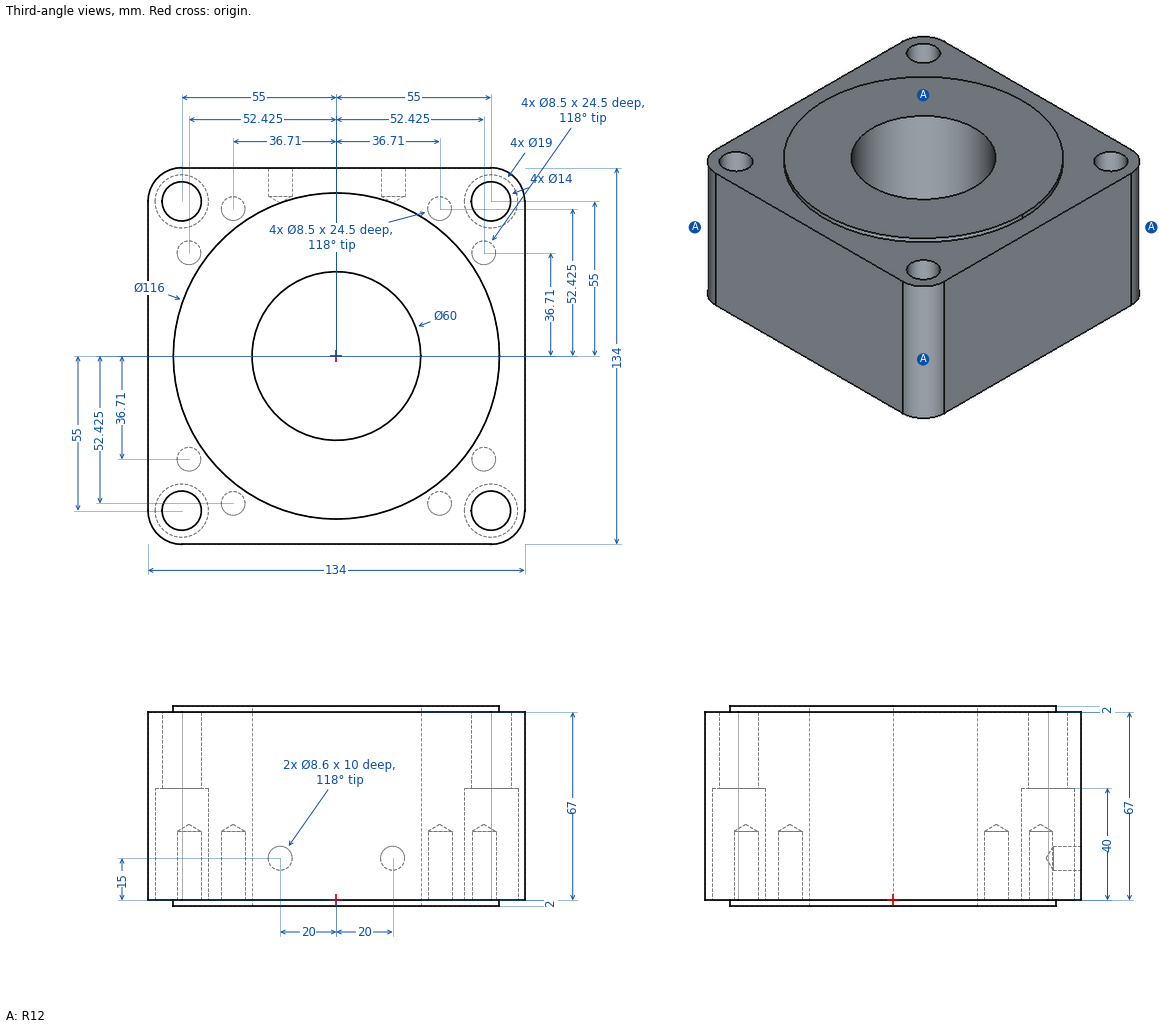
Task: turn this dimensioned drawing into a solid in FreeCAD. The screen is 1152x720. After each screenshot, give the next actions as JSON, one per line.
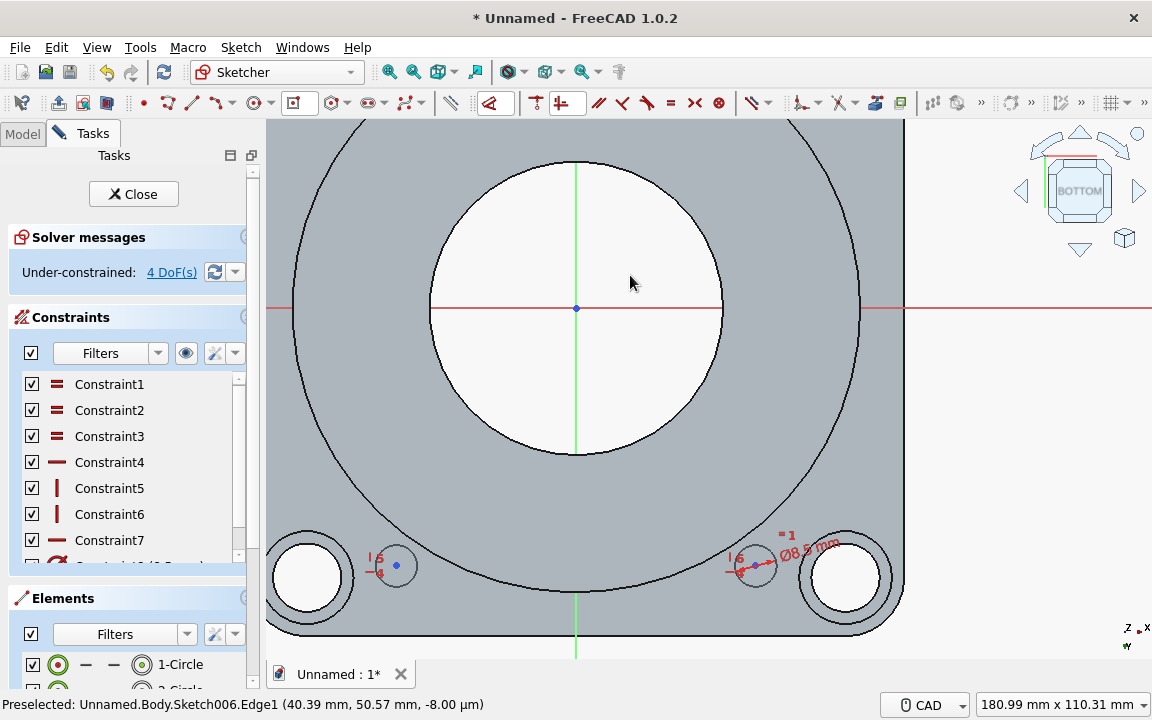
{"action": "left_click", "coordinate": [756, 566]}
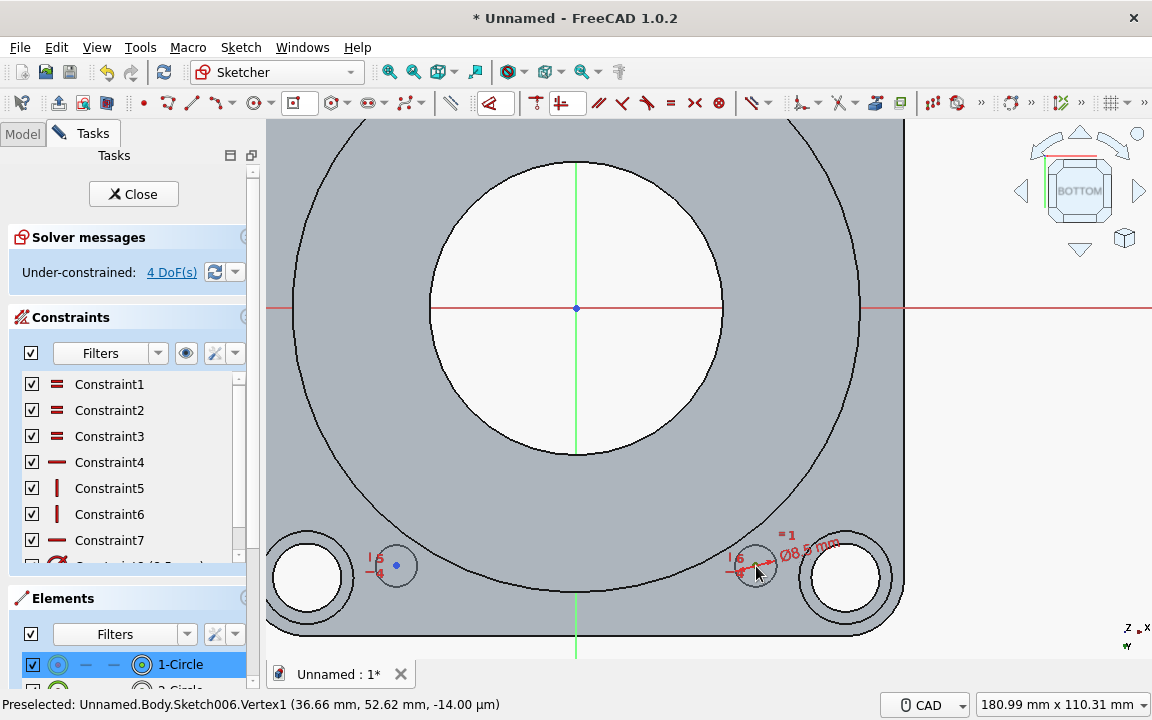
{"action": "key", "text": "l"}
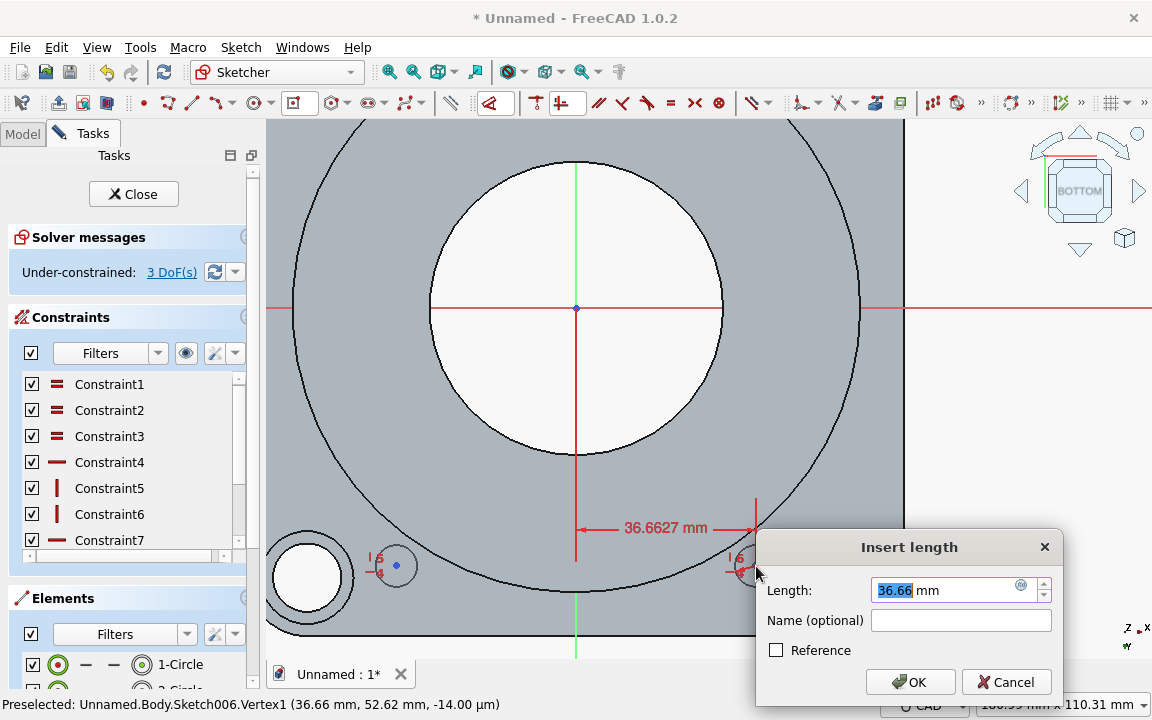
{"action": "type", "text": "36.71"}
{"action": "key", "text": "Return"}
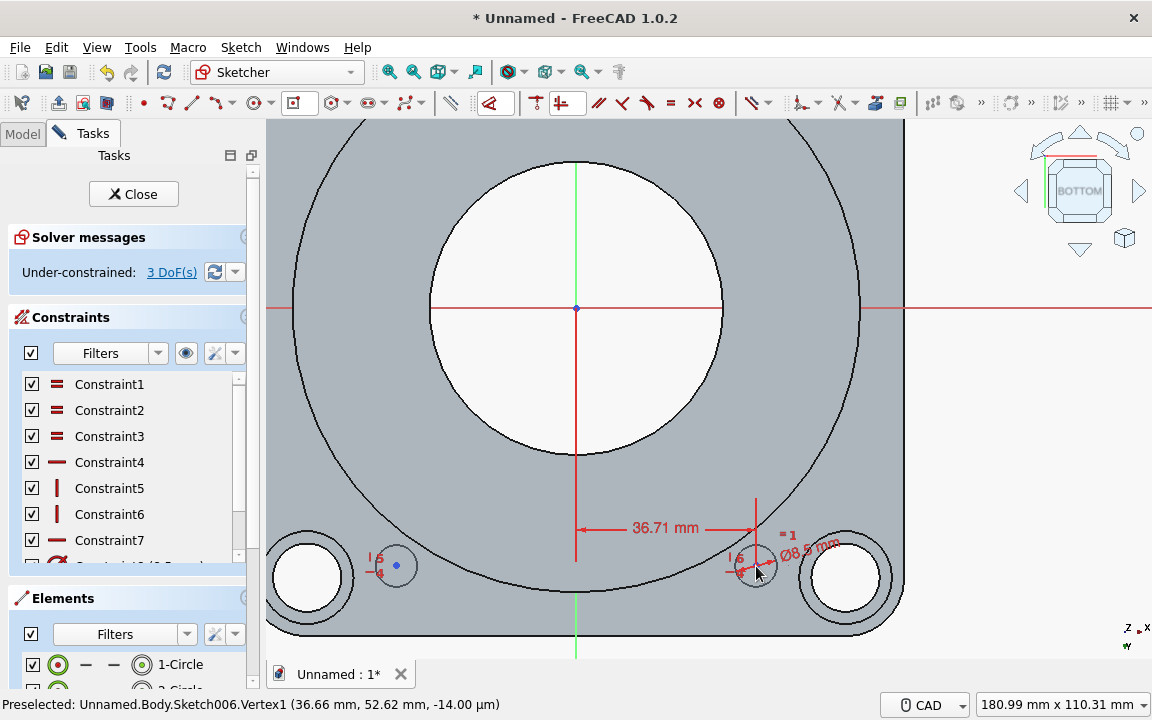
{"action": "left_click", "coordinate": [396, 566]}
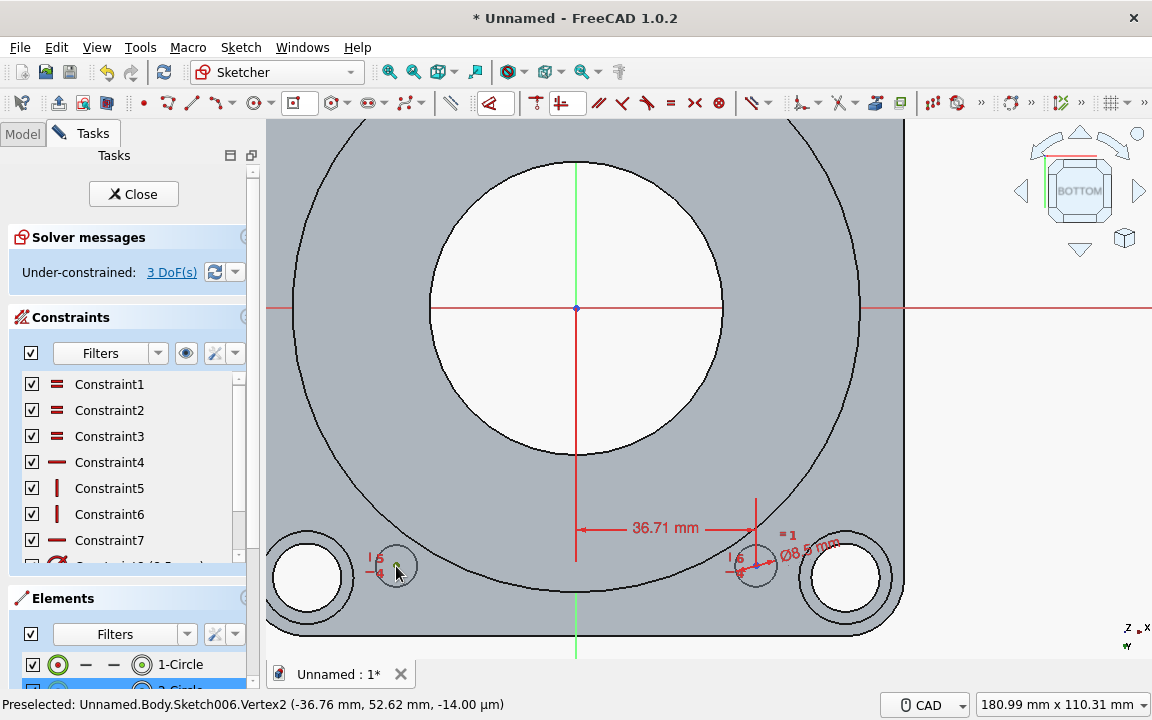
{"action": "key", "text": "l"}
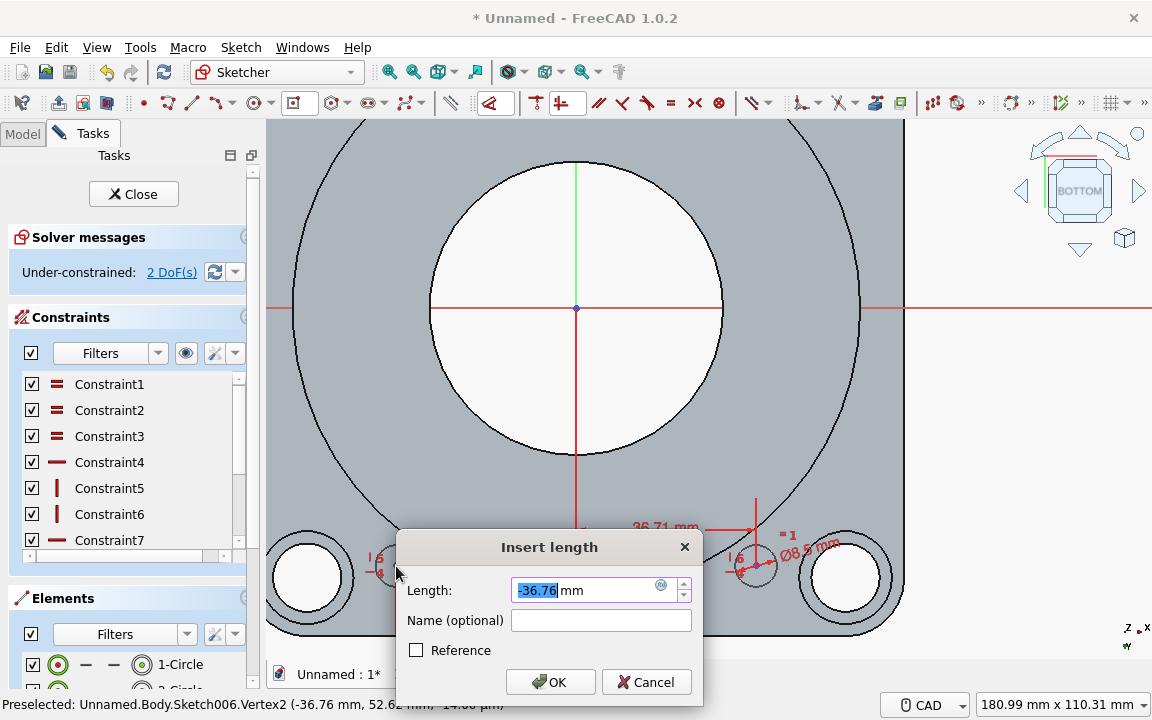
{"action": "type", "text": "-36.71"}
{"action": "key", "text": "Return"}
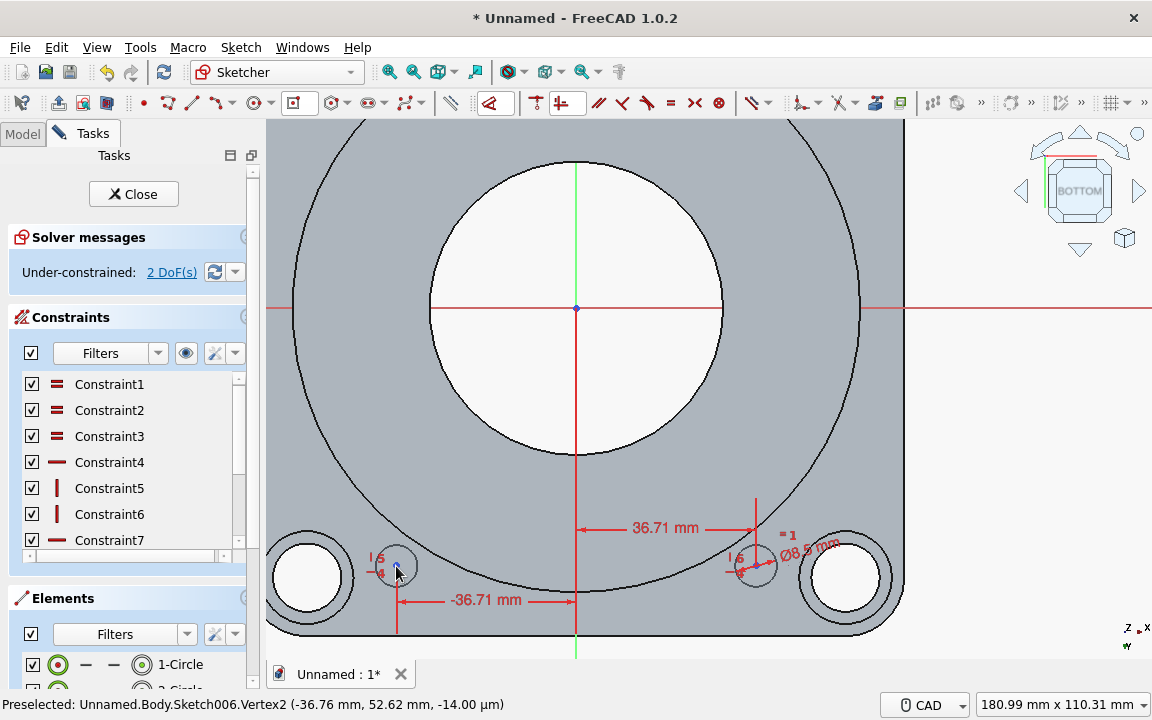
{"action": "left_click", "coordinate": [756, 566]}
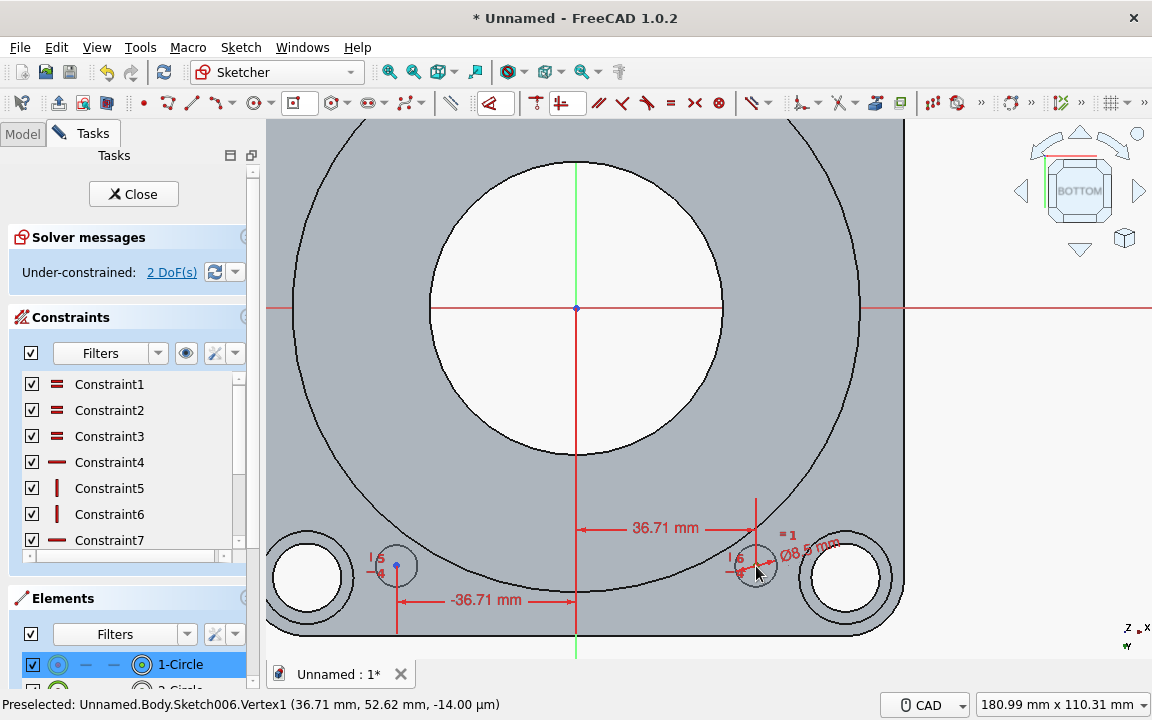
{"action": "key", "text": "i"}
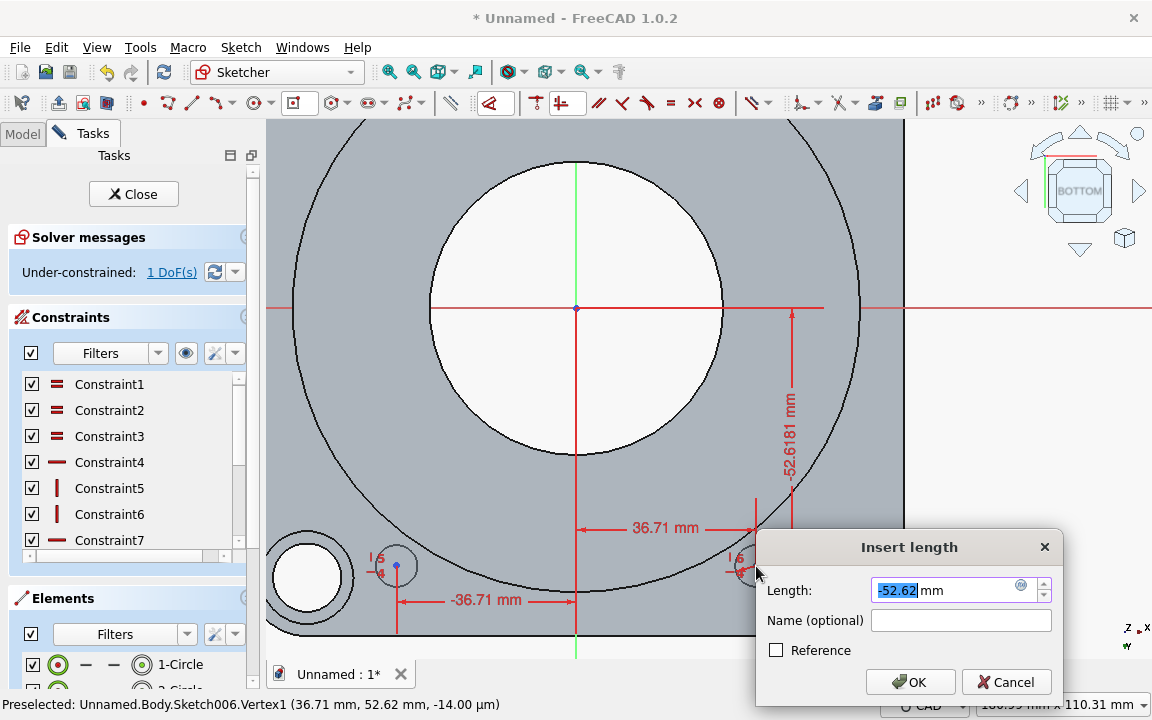
{"action": "type", "text": "-52.425"}
{"action": "key", "text": "Return"}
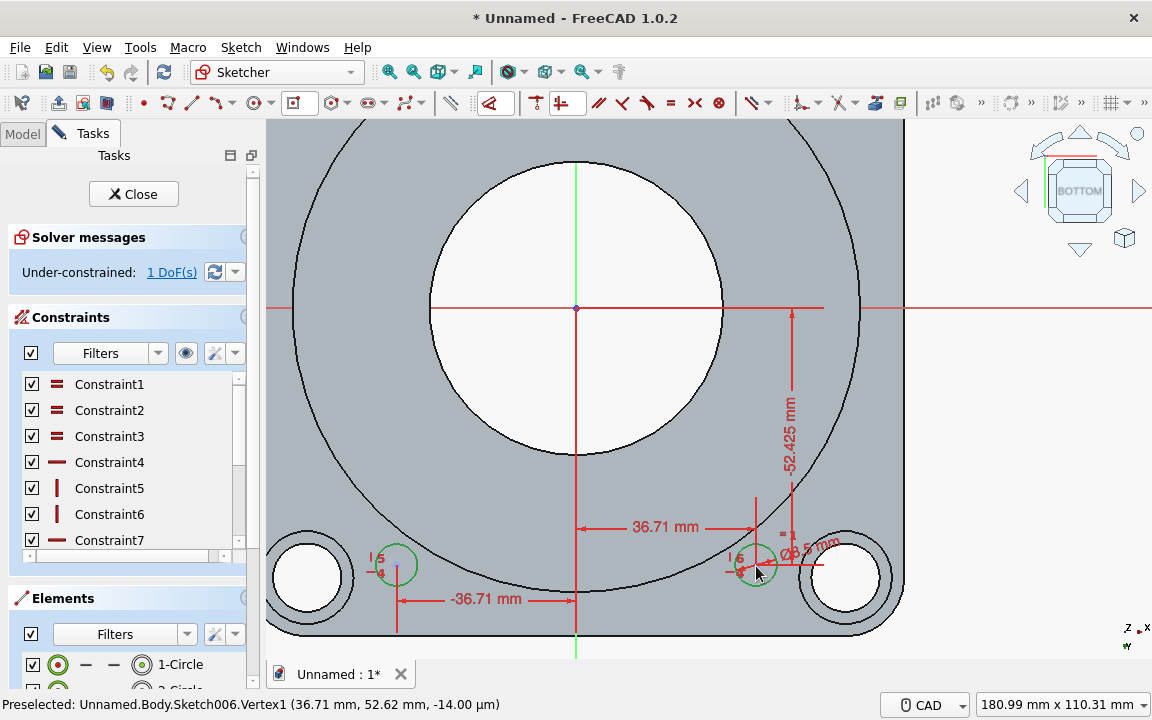
{"action": "scroll", "coordinate": [771, 553], "scroll_direction": "down", "scroll_amount": 2}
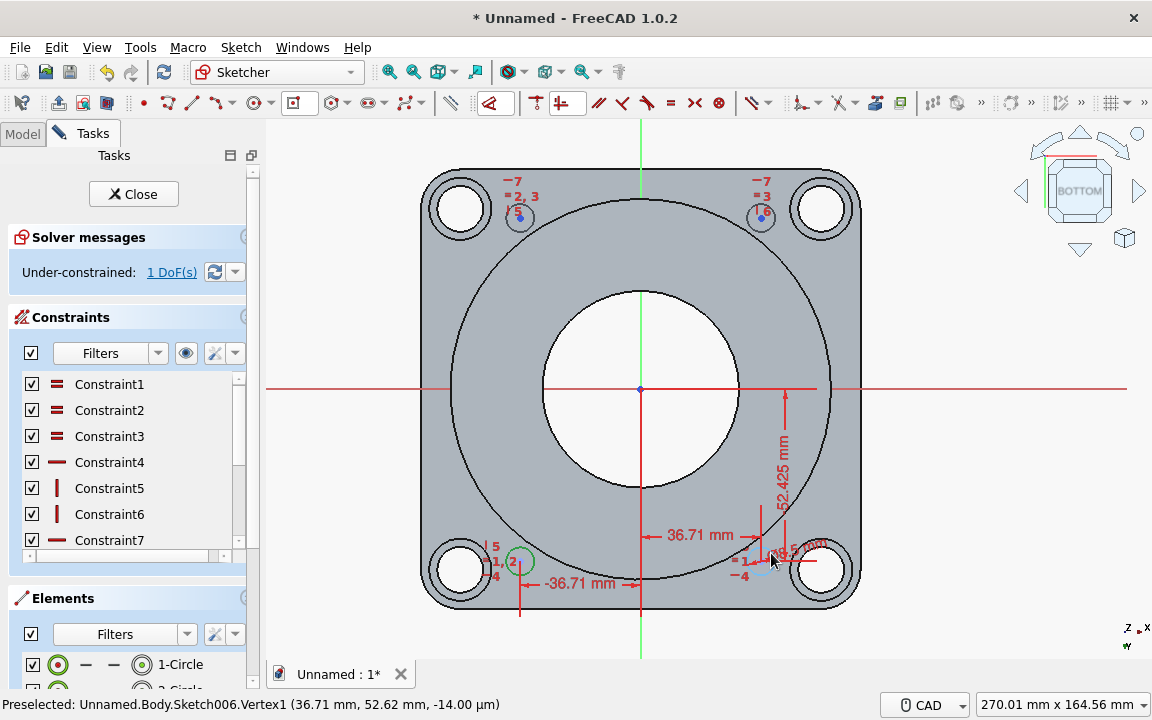
{"action": "left_click", "coordinate": [520, 218]}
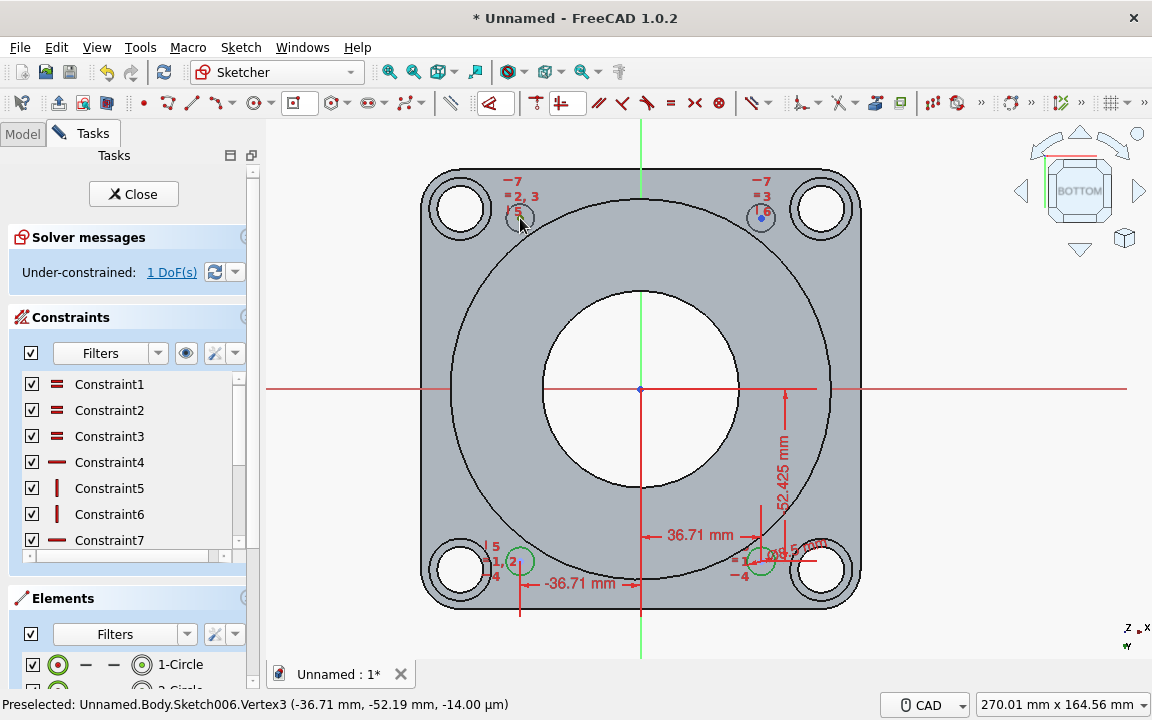
{"action": "left_click", "coordinate": [508, 104]}